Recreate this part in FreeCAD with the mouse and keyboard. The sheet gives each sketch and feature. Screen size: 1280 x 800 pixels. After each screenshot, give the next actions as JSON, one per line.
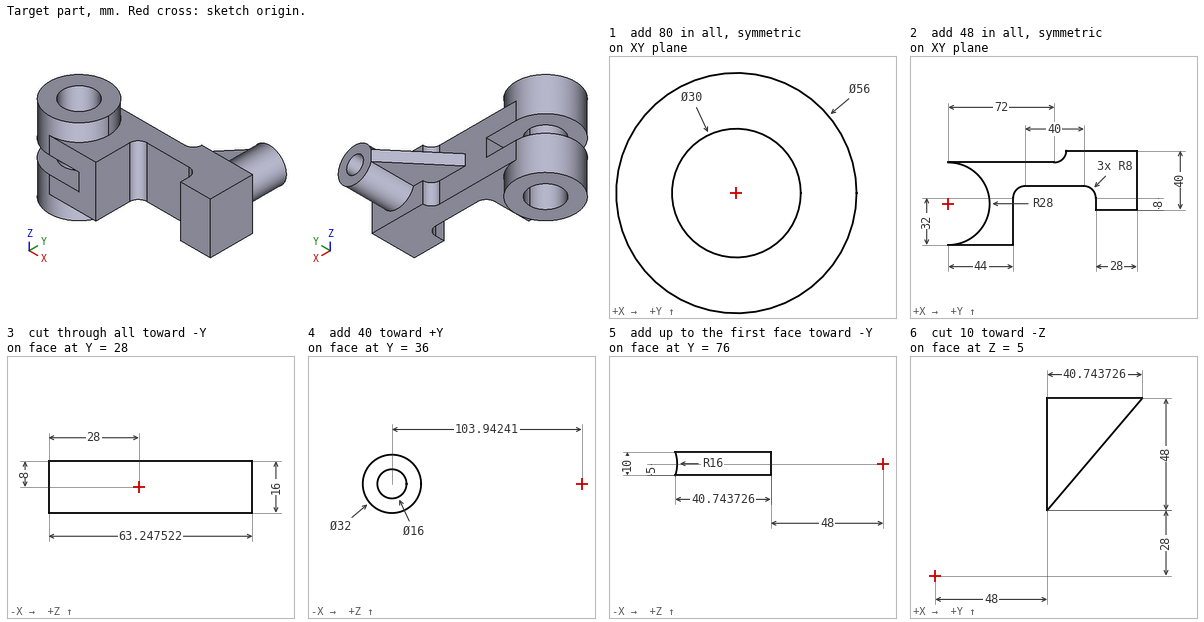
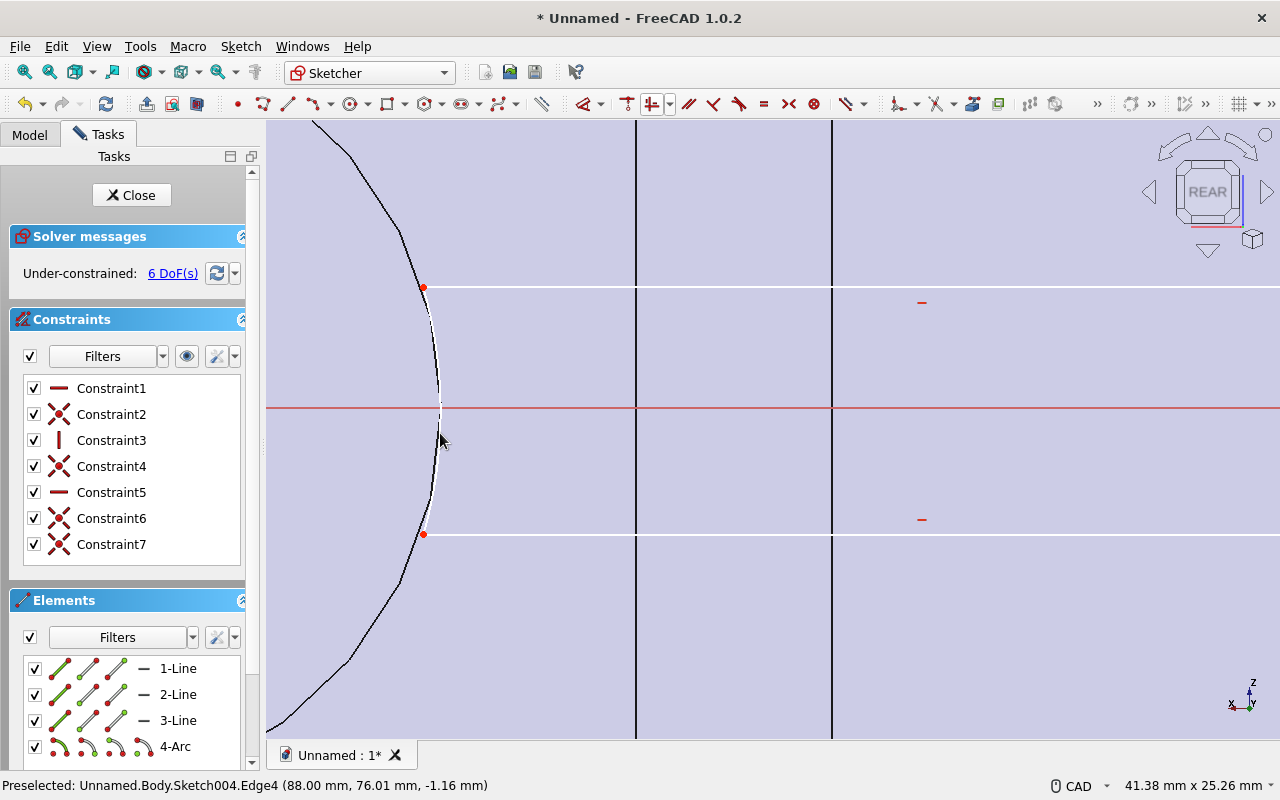
{"action": "scroll", "coordinate": [441, 437], "scroll_direction": "down", "scroll_amount": 7}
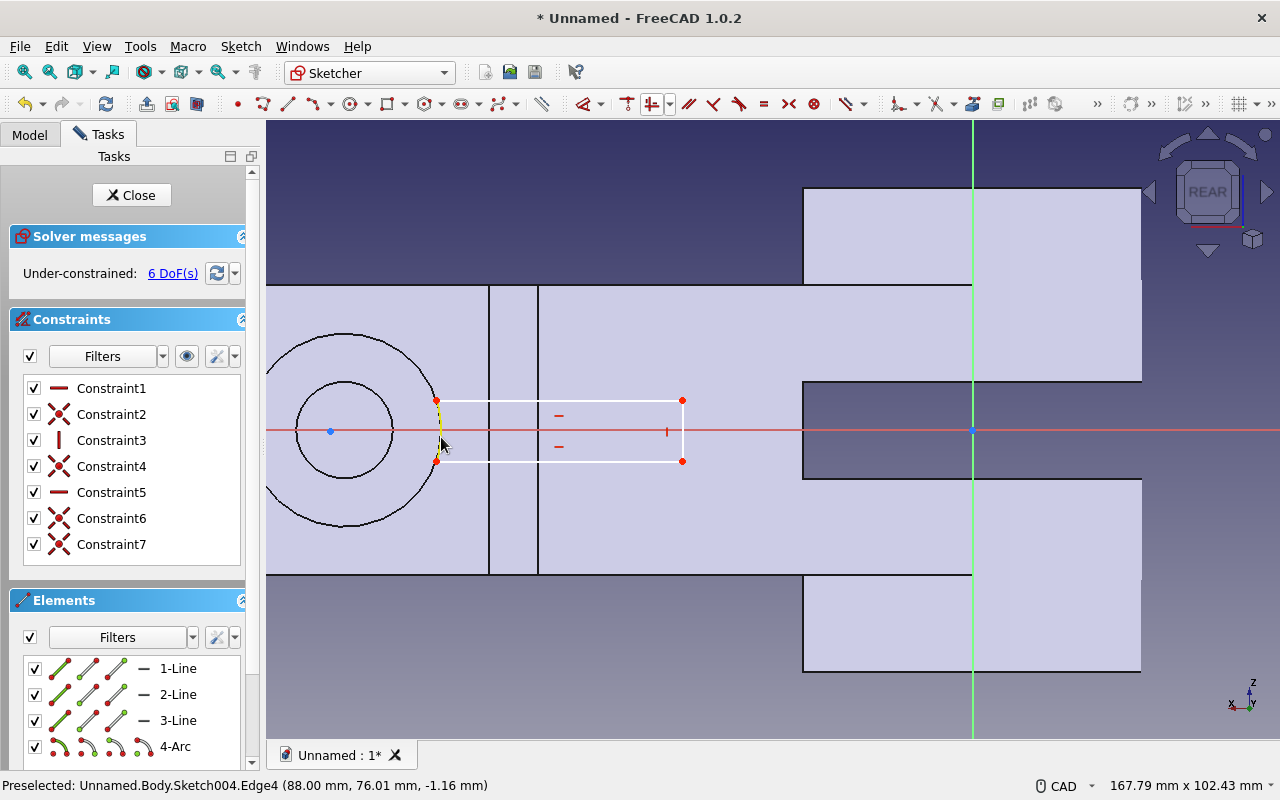
{"action": "left_click", "coordinate": [330, 431]}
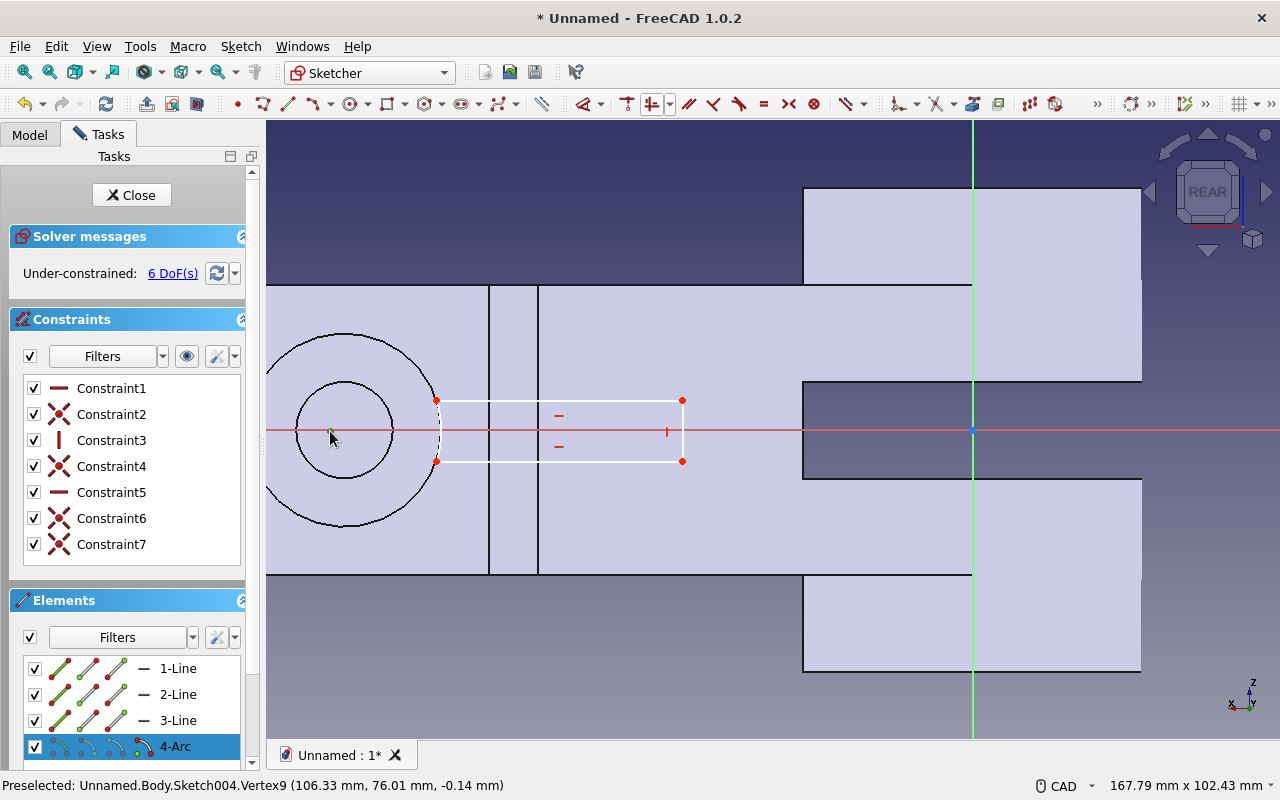
{"action": "left_click", "coordinate": [353, 430]}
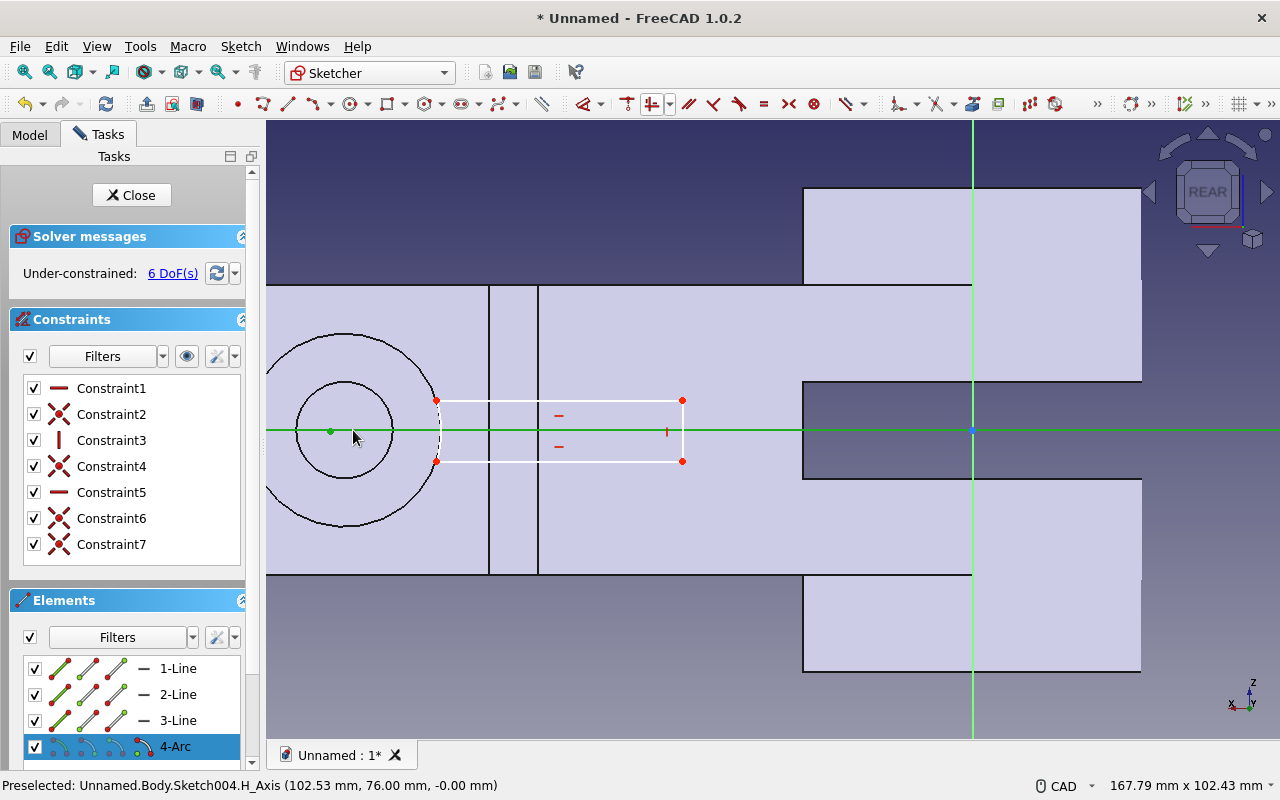
{"action": "left_click", "coordinate": [627, 104]}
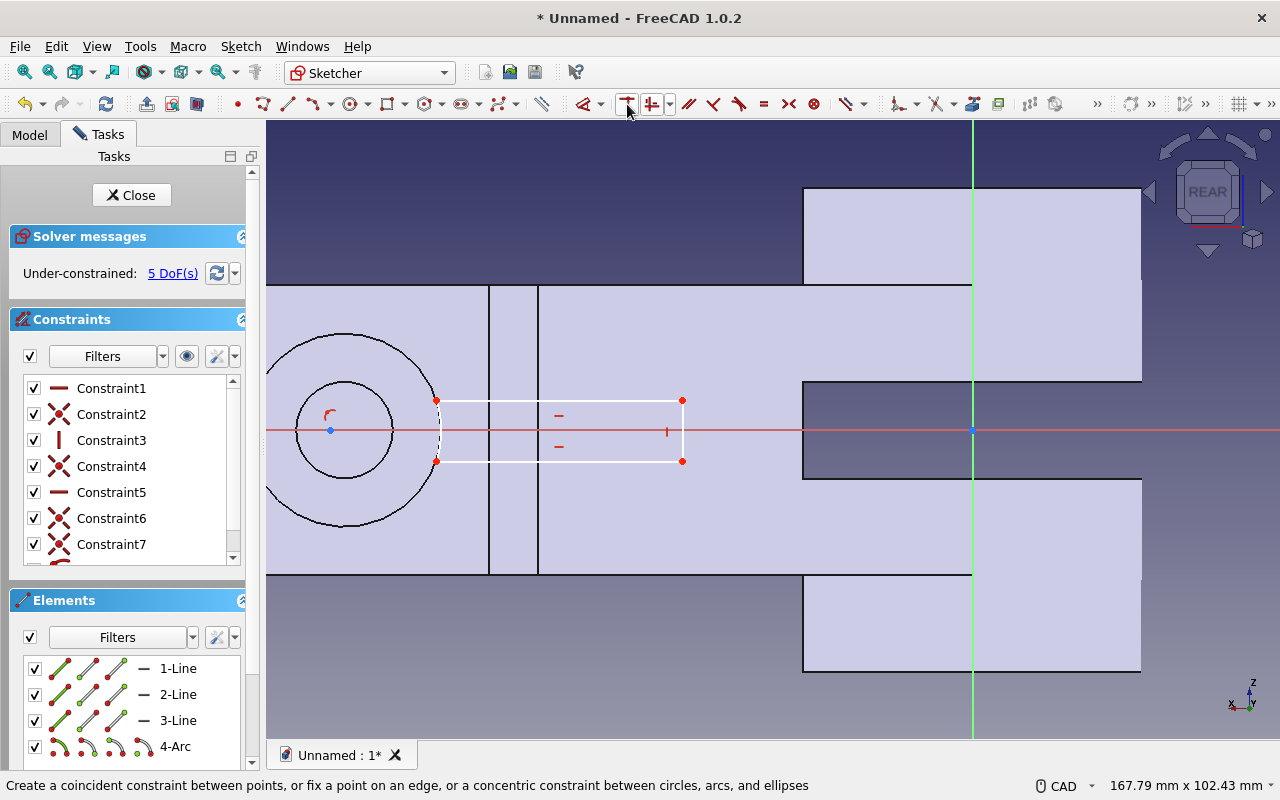
{"action": "key", "text": "d"}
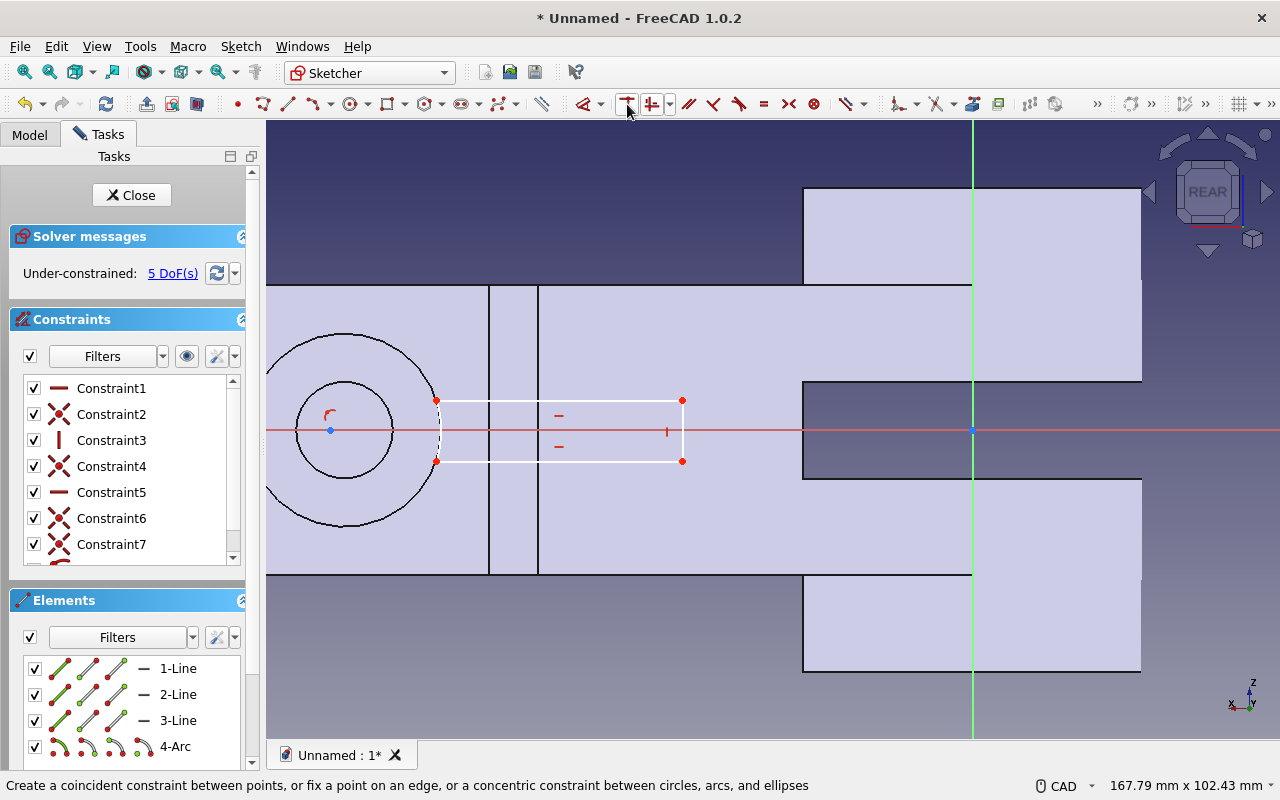
{"action": "left_click", "coordinate": [440, 443]}
{"action": "left_click", "coordinate": [472, 447]}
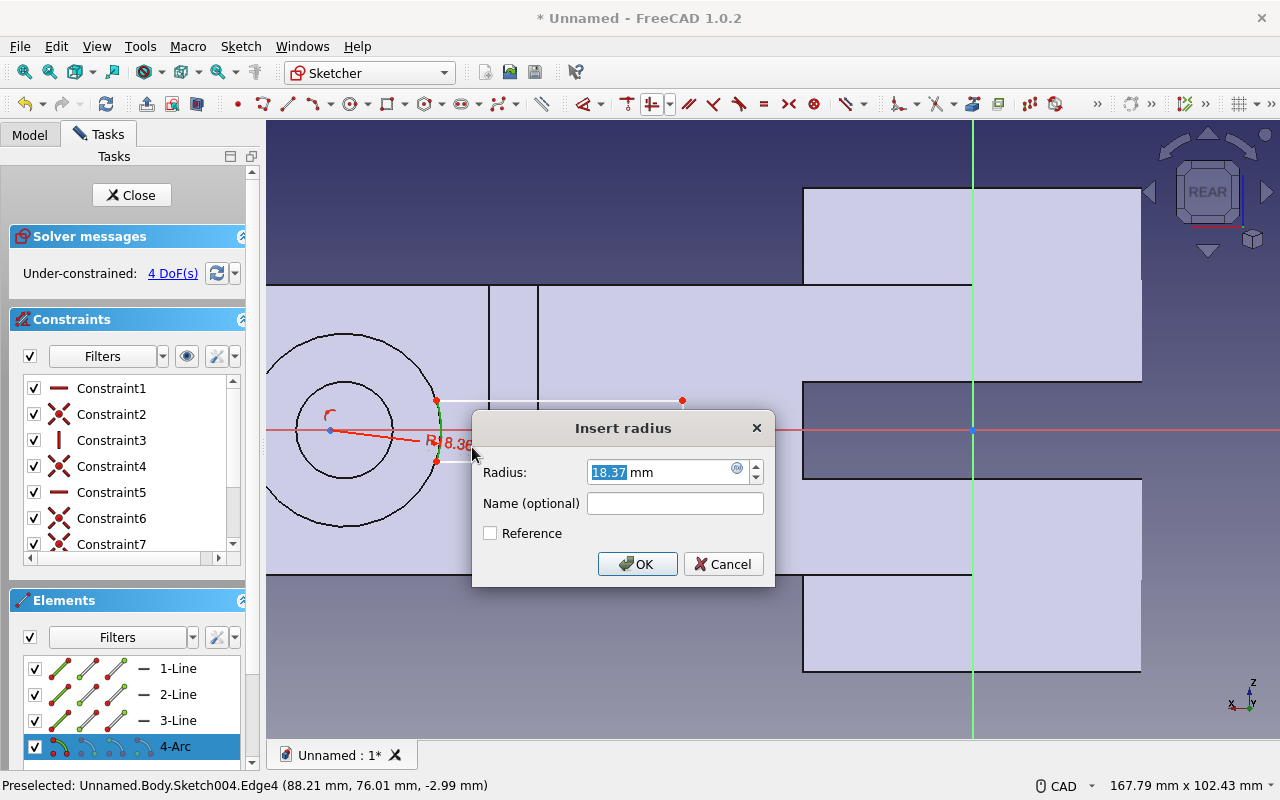
{"action": "type", "text": "16"}
{"action": "key", "text": "Return"}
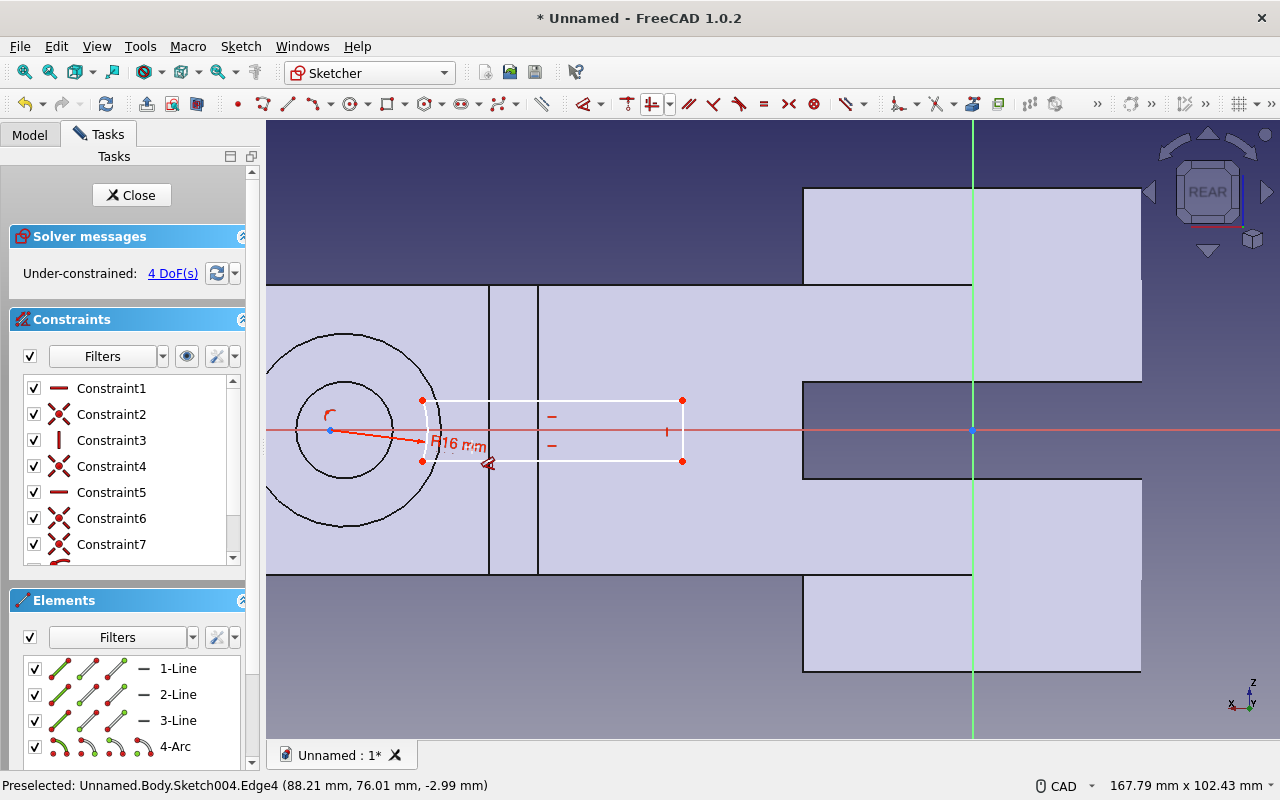
{"action": "left_click", "coordinate": [683, 443]}
{"action": "left_click", "coordinate": [649, 417]}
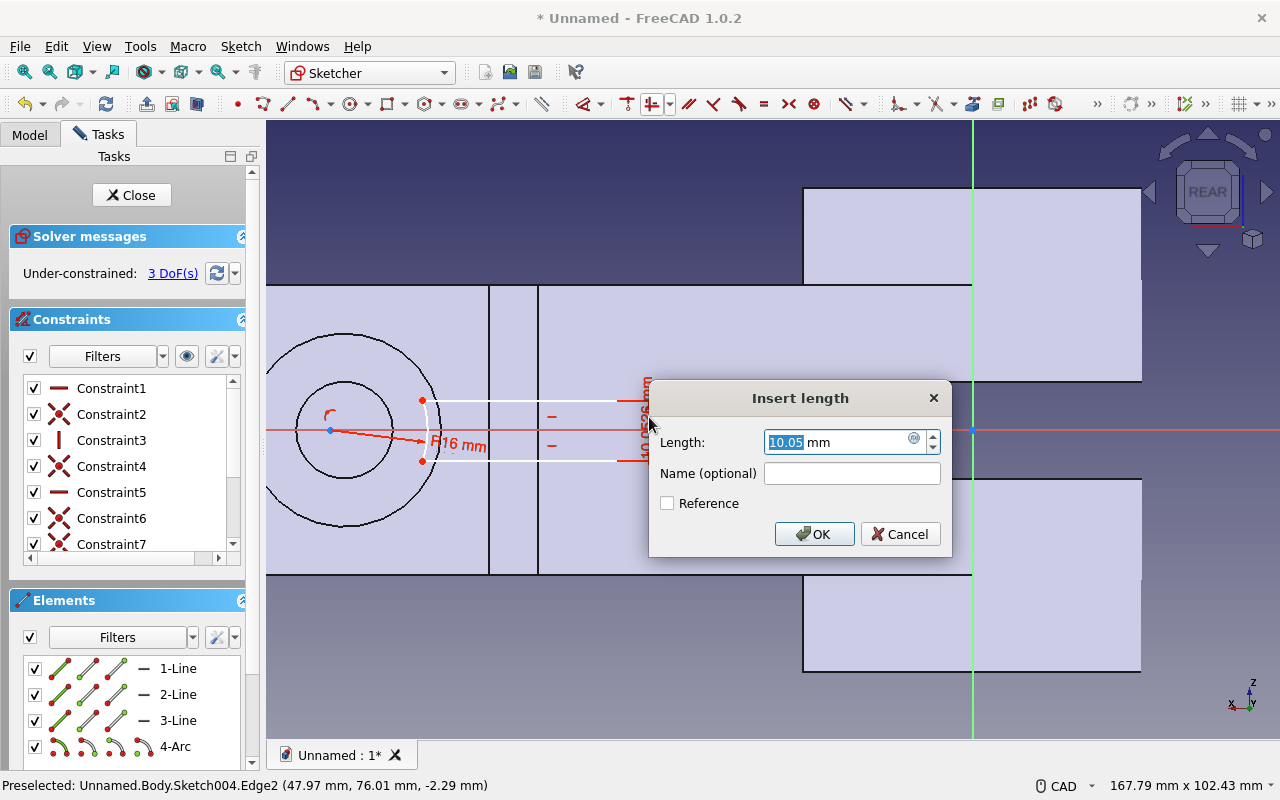
{"action": "type", "text": "10"}
{"action": "key", "text": "Return"}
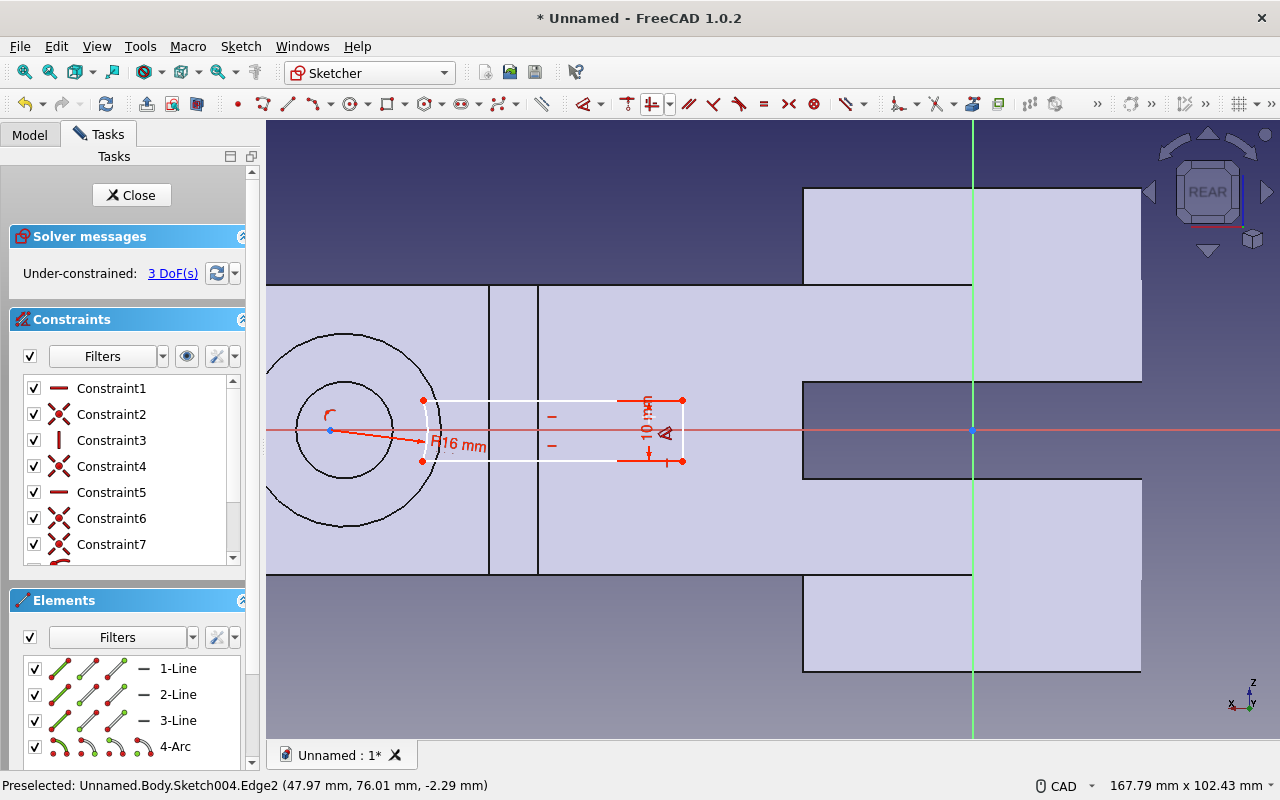
{"action": "scroll", "coordinate": [422, 461], "scroll_direction": "up", "scroll_amount": 2}